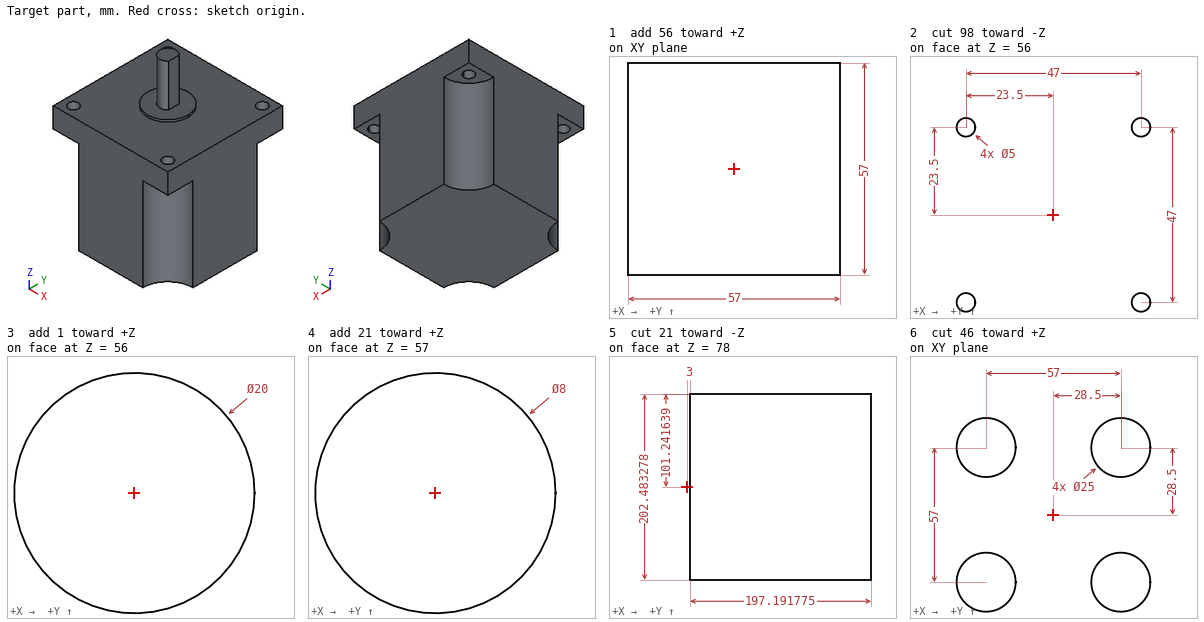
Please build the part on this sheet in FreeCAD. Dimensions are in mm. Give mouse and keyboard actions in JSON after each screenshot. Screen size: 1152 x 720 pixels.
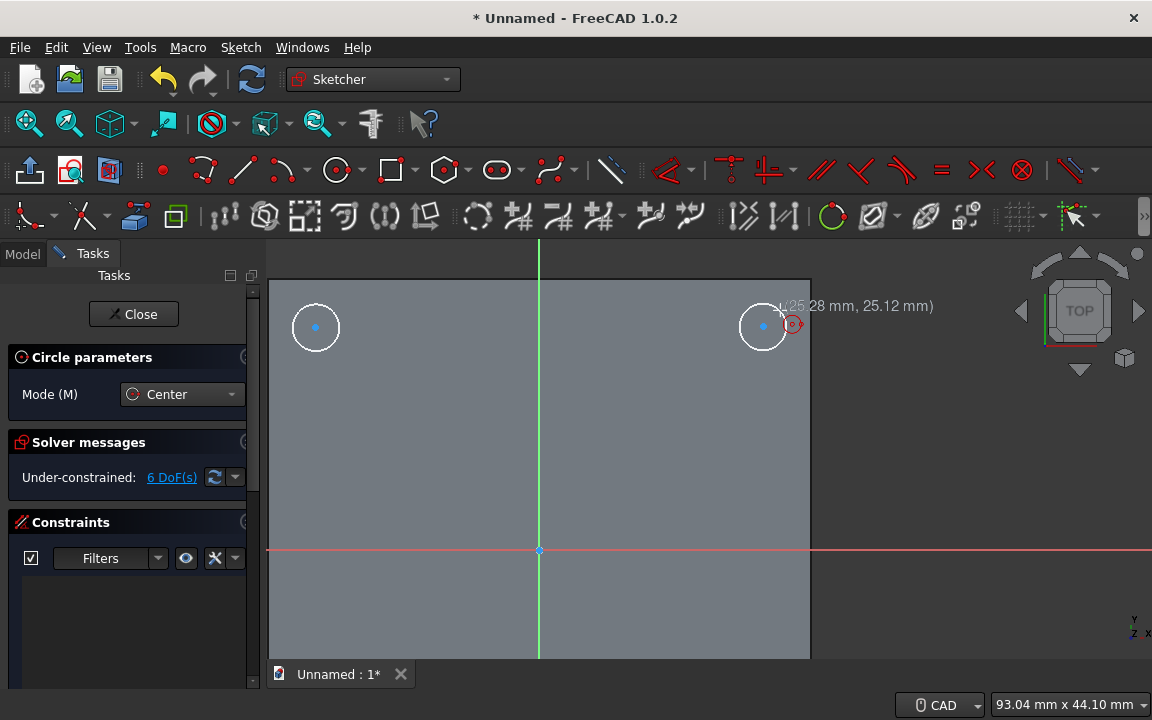
{"action": "scroll", "coordinate": [764, 326], "scroll_direction": "down", "scroll_amount": 3}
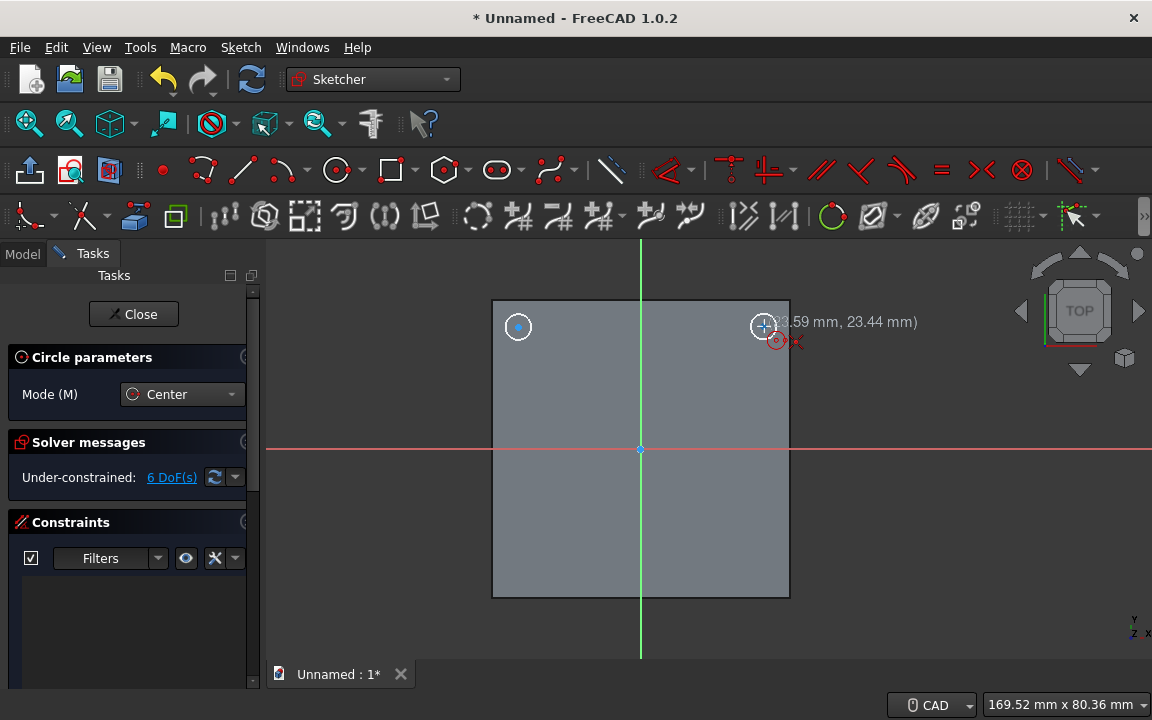
{"action": "scroll", "coordinate": [764, 572], "scroll_direction": "up", "scroll_amount": 3}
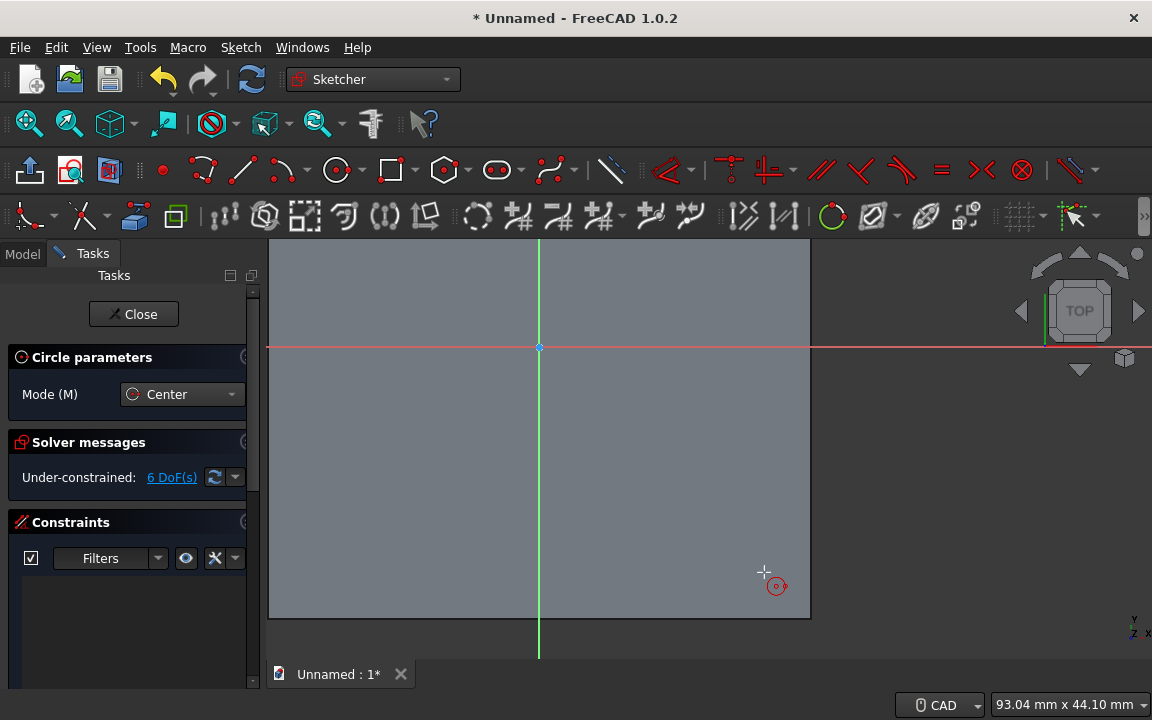
{"action": "left_click", "coordinate": [763, 571]}
{"action": "left_click", "coordinate": [780, 554]}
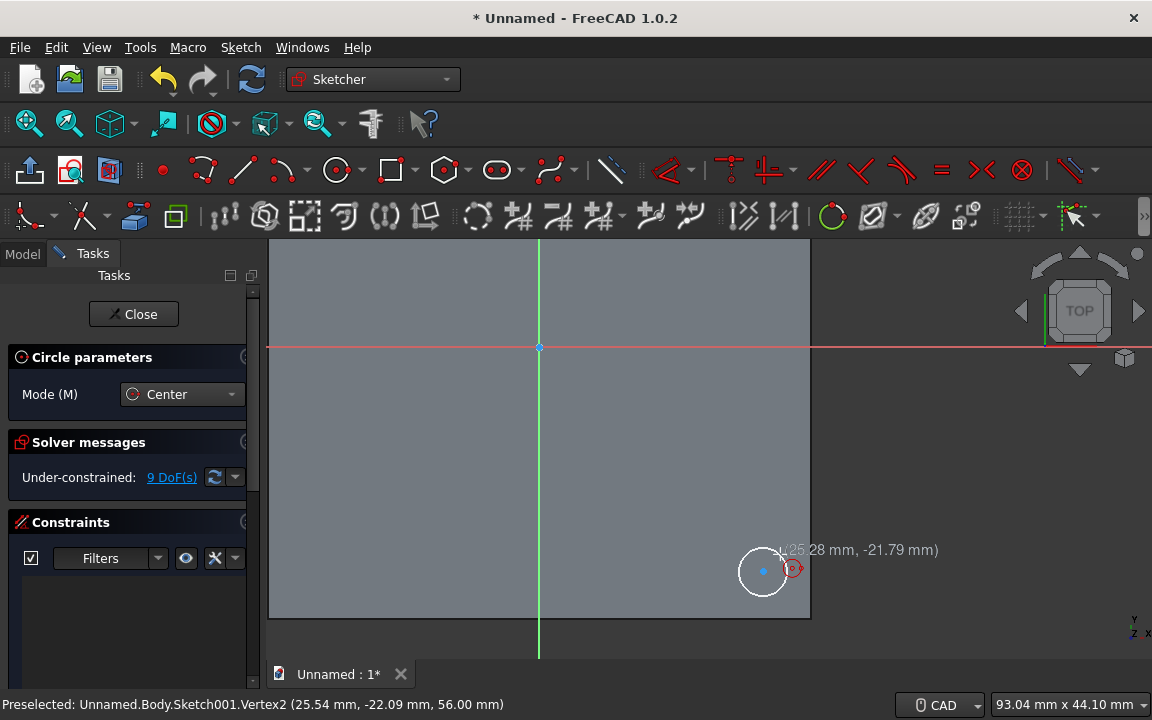
{"action": "left_click", "coordinate": [316, 571]}
{"action": "left_click", "coordinate": [332, 554]}
{"action": "key", "text": "Escape"}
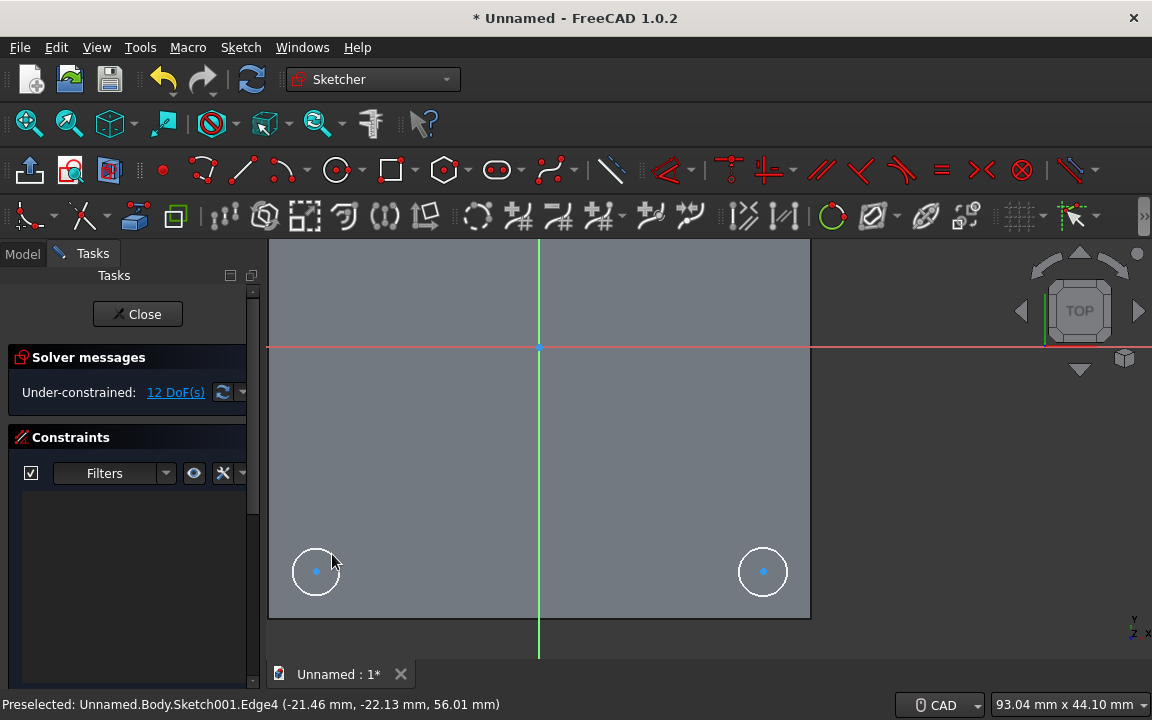
{"action": "scroll", "coordinate": [764, 572], "scroll_direction": "down", "scroll_amount": 3}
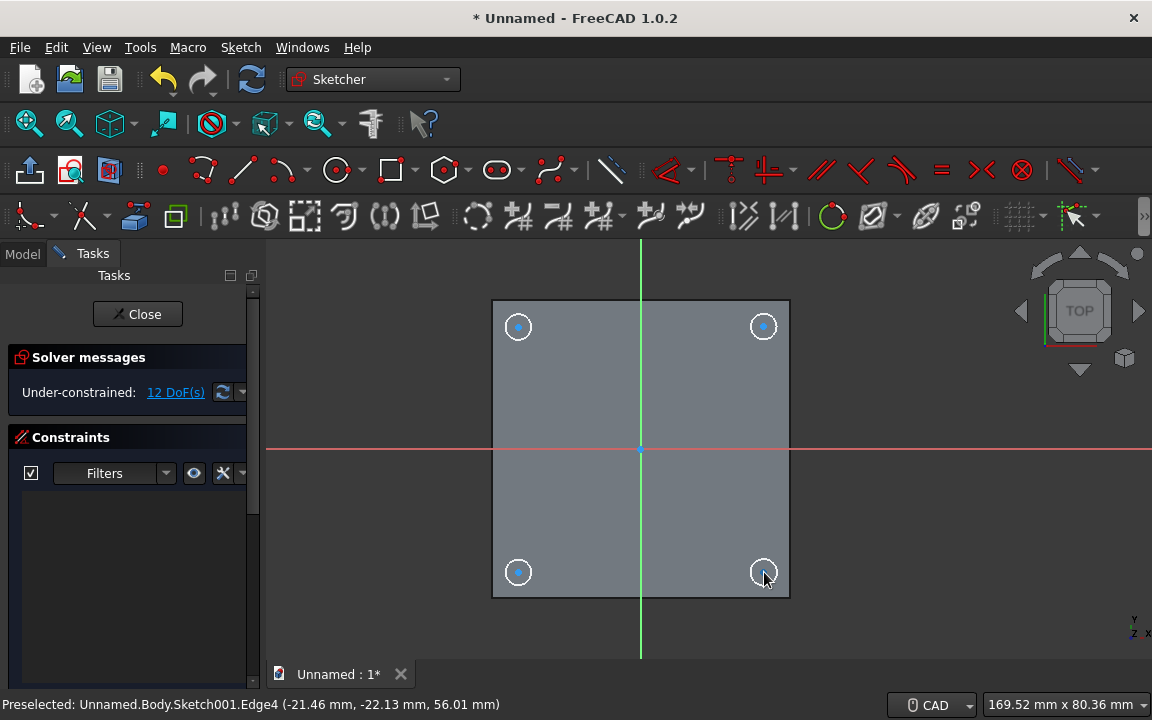
{"action": "left_click", "coordinate": [527, 318]}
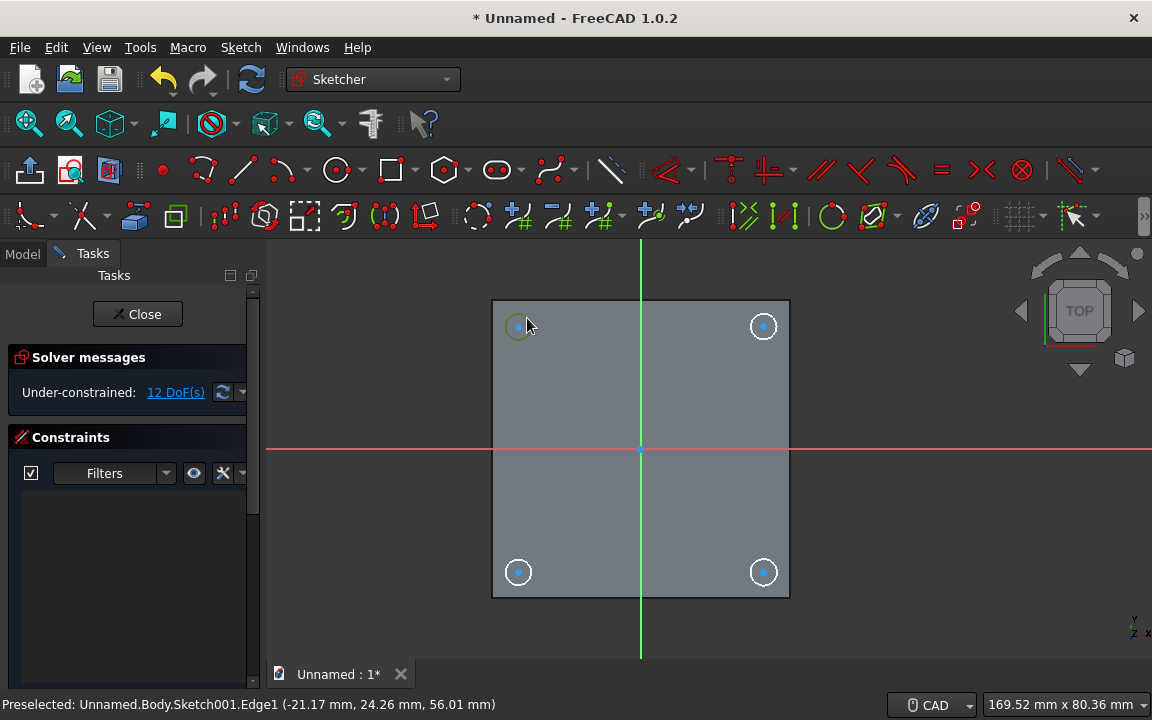
{"action": "left_click", "coordinate": [773, 318]}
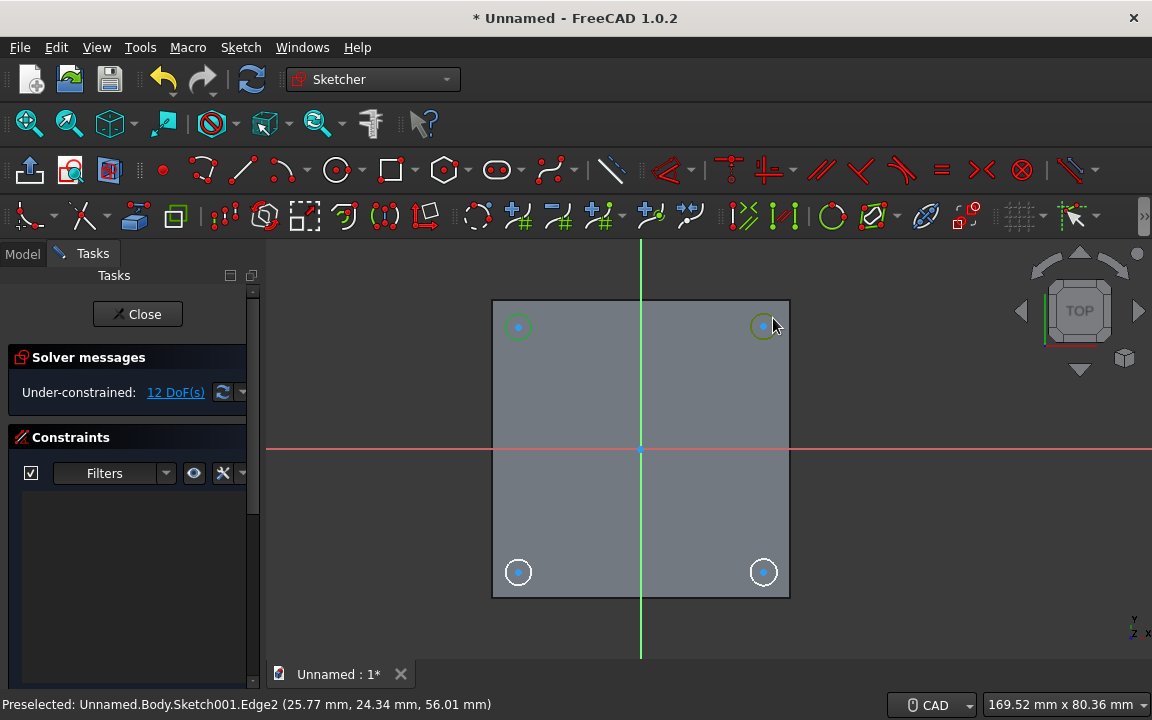
{"action": "left_click", "coordinate": [773, 563]}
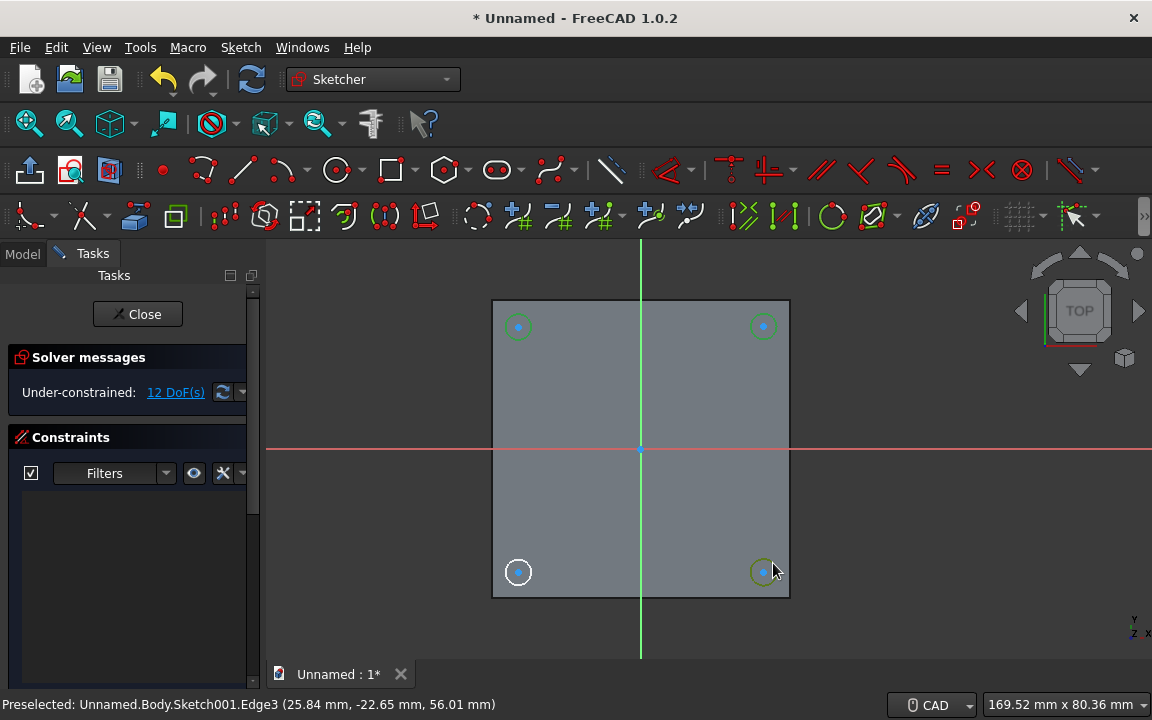
{"action": "left_click", "coordinate": [527, 563]}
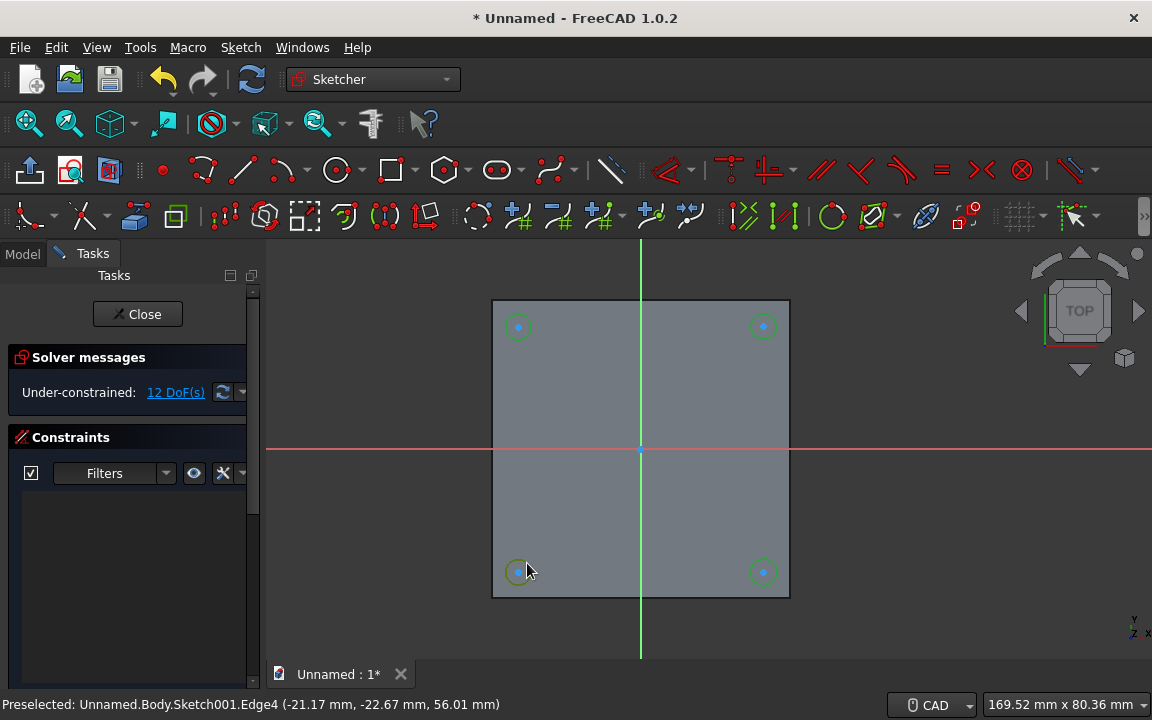
{"action": "left_click", "coordinate": [942, 170]}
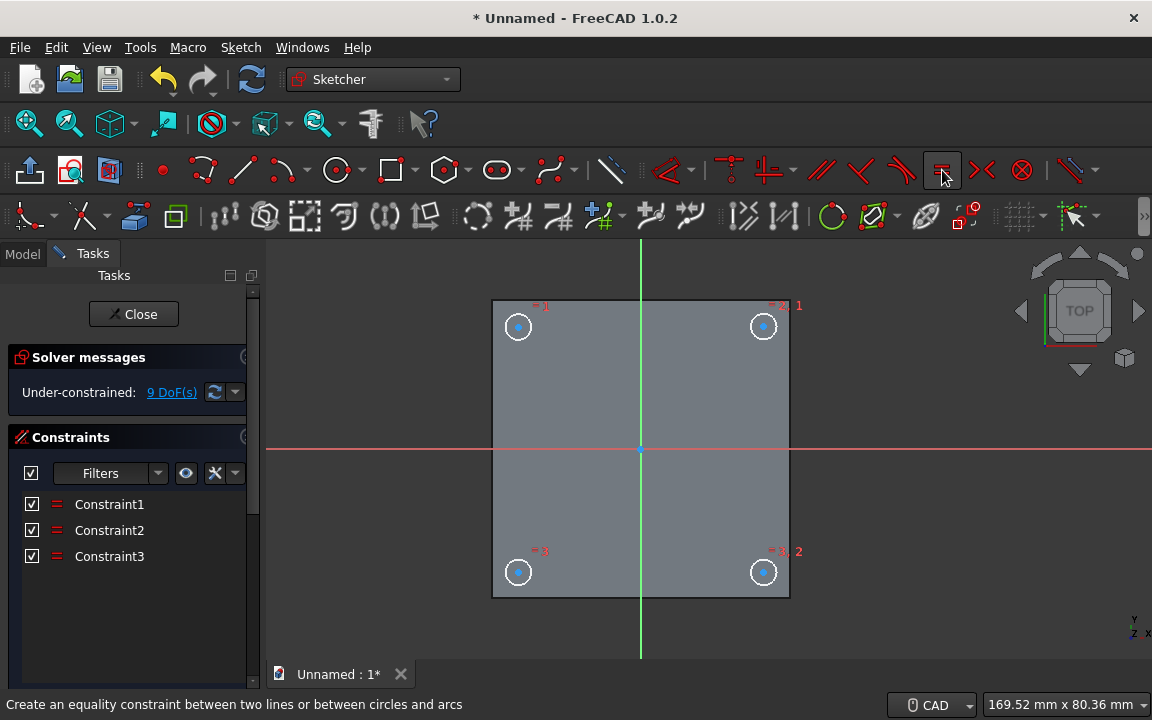
{"action": "left_click", "coordinate": [518, 327]}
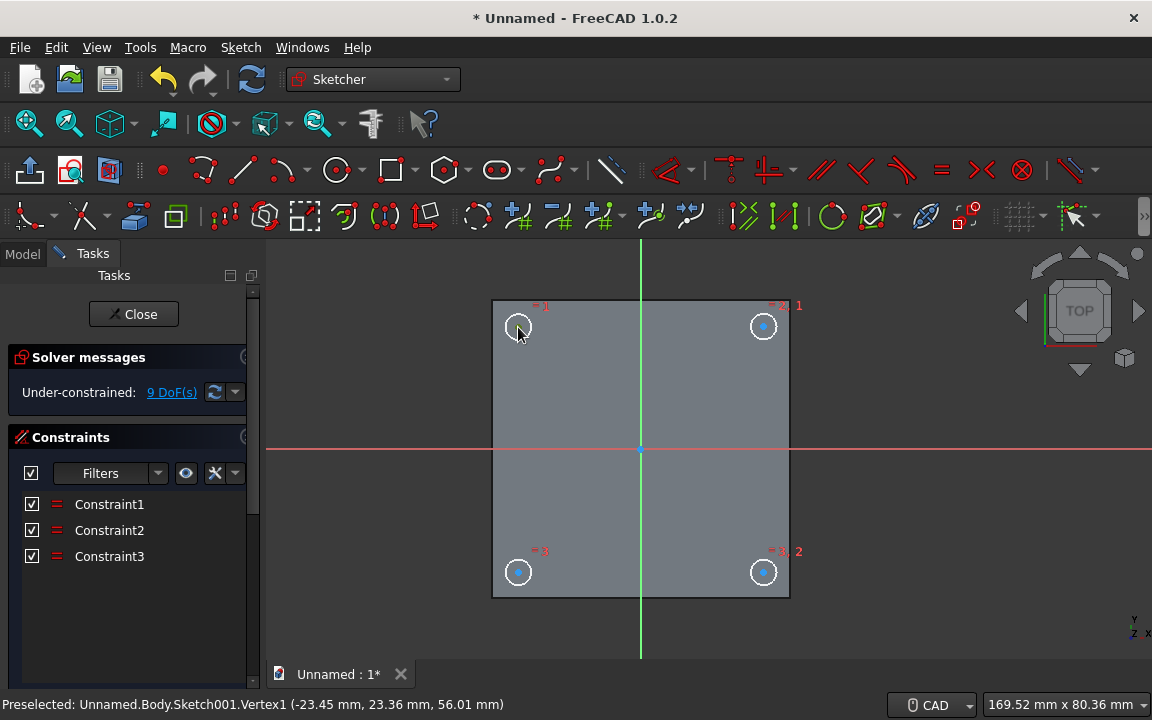
{"action": "left_click", "coordinate": [764, 327]}